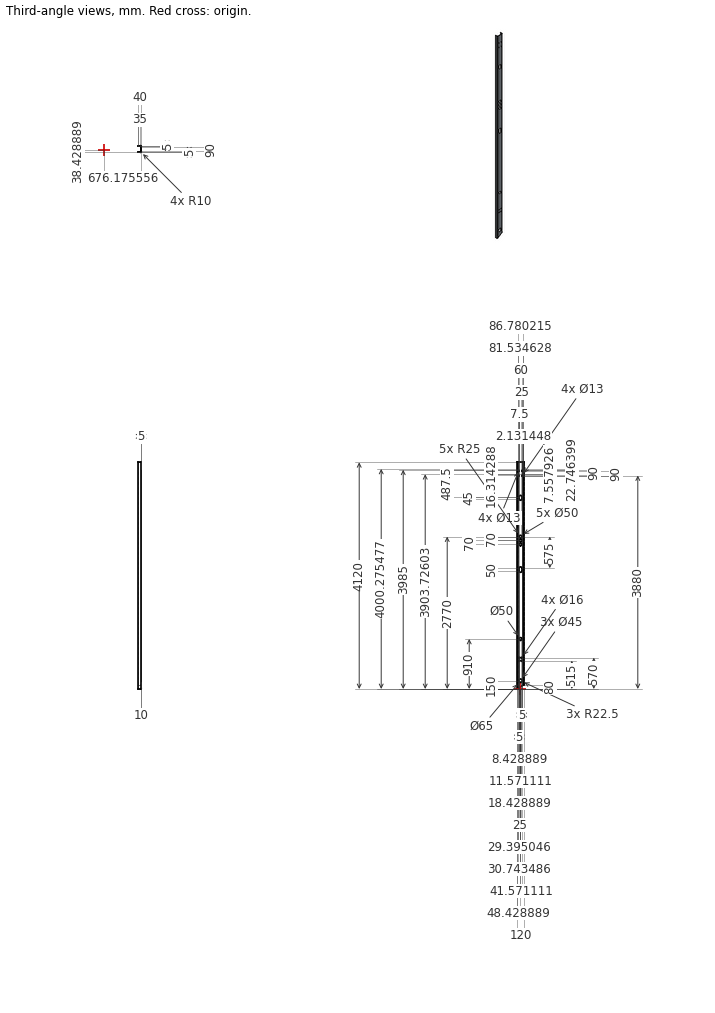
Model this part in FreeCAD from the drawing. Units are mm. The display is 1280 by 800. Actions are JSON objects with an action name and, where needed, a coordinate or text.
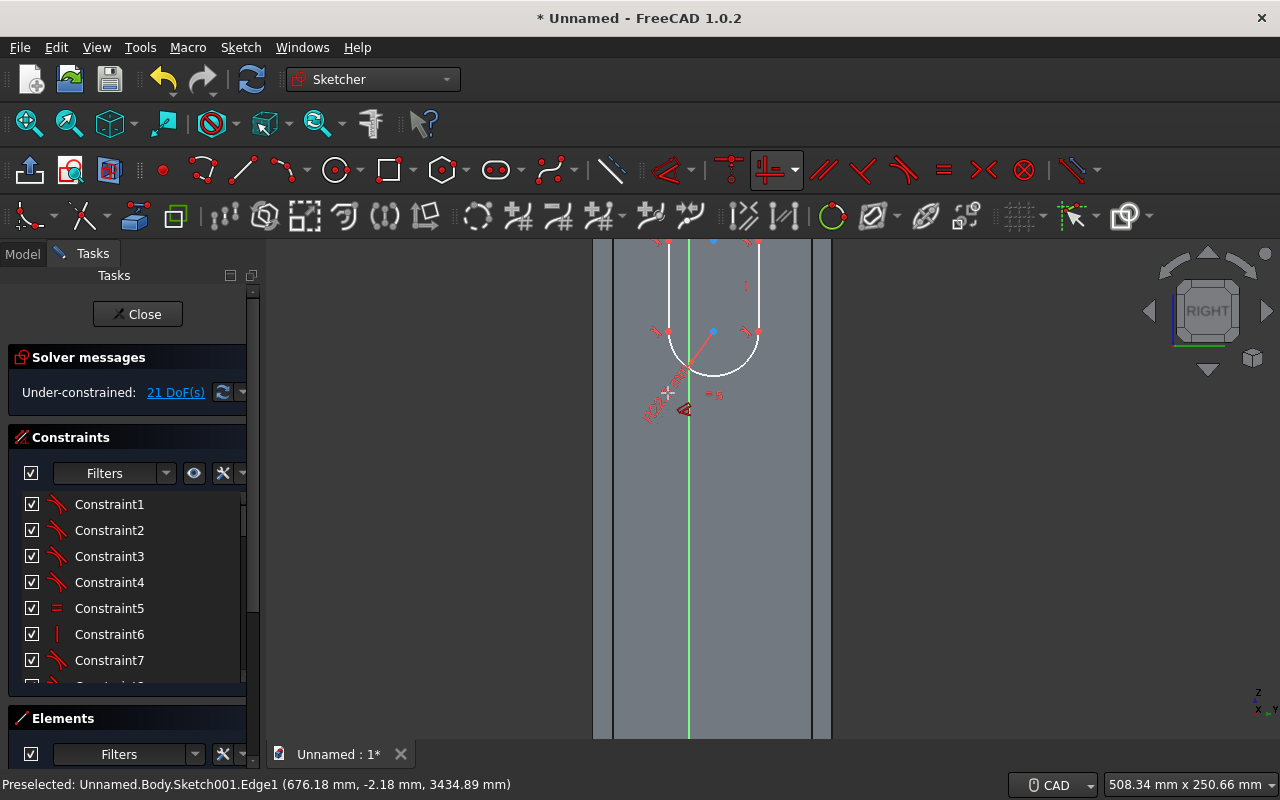
{"action": "scroll", "coordinate": [704, 372], "scroll_direction": "down", "scroll_amount": 16}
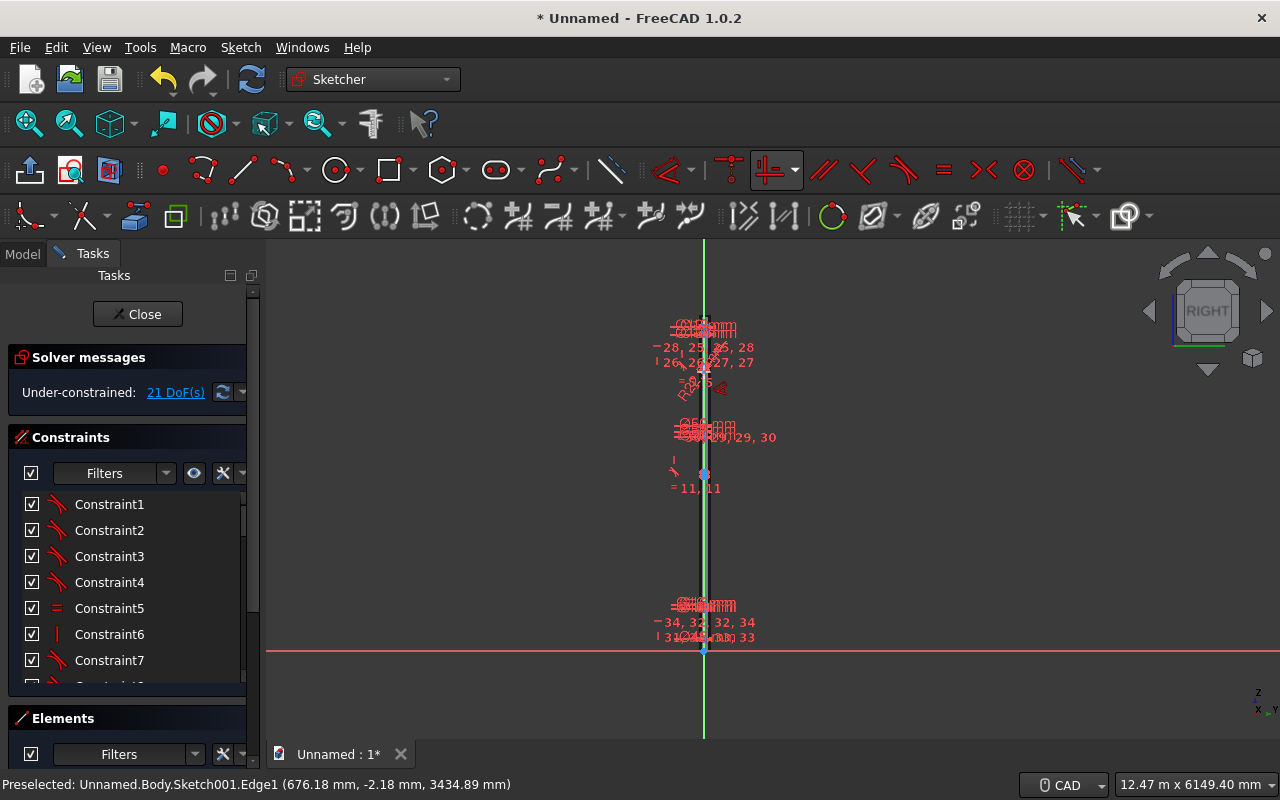
{"action": "scroll", "coordinate": [706, 479], "scroll_direction": "up", "scroll_amount": 15}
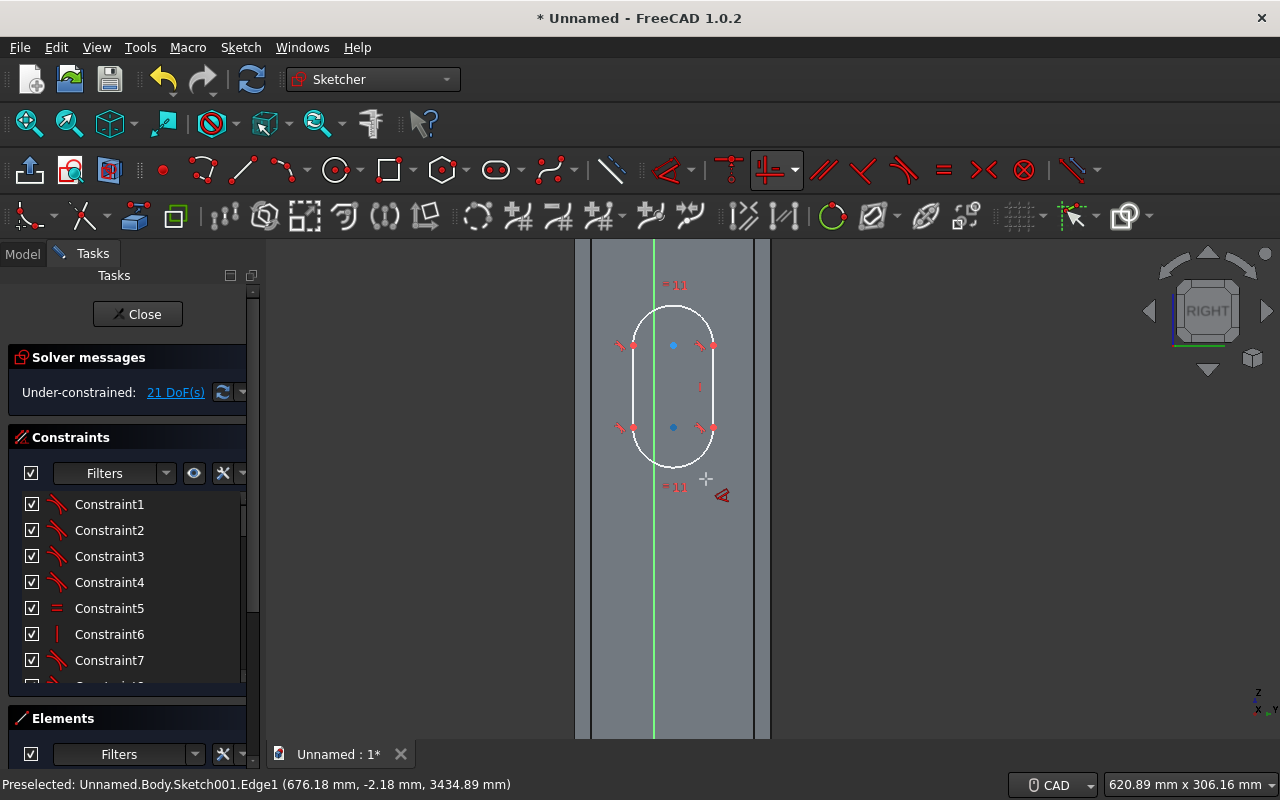
{"action": "left_click", "coordinate": [697, 460]}
{"action": "left_click", "coordinate": [716, 486]}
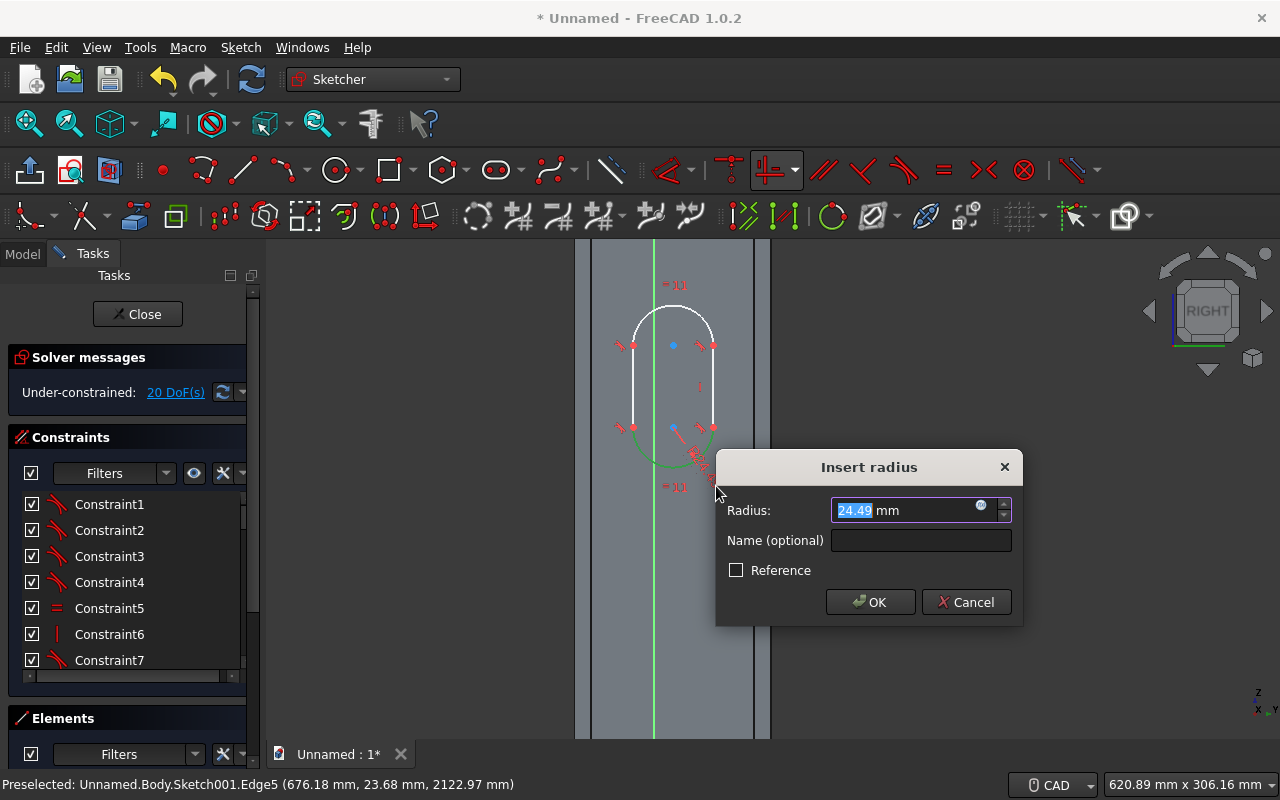
{"action": "type", "text": "25"}
{"action": "key", "text": "Return"}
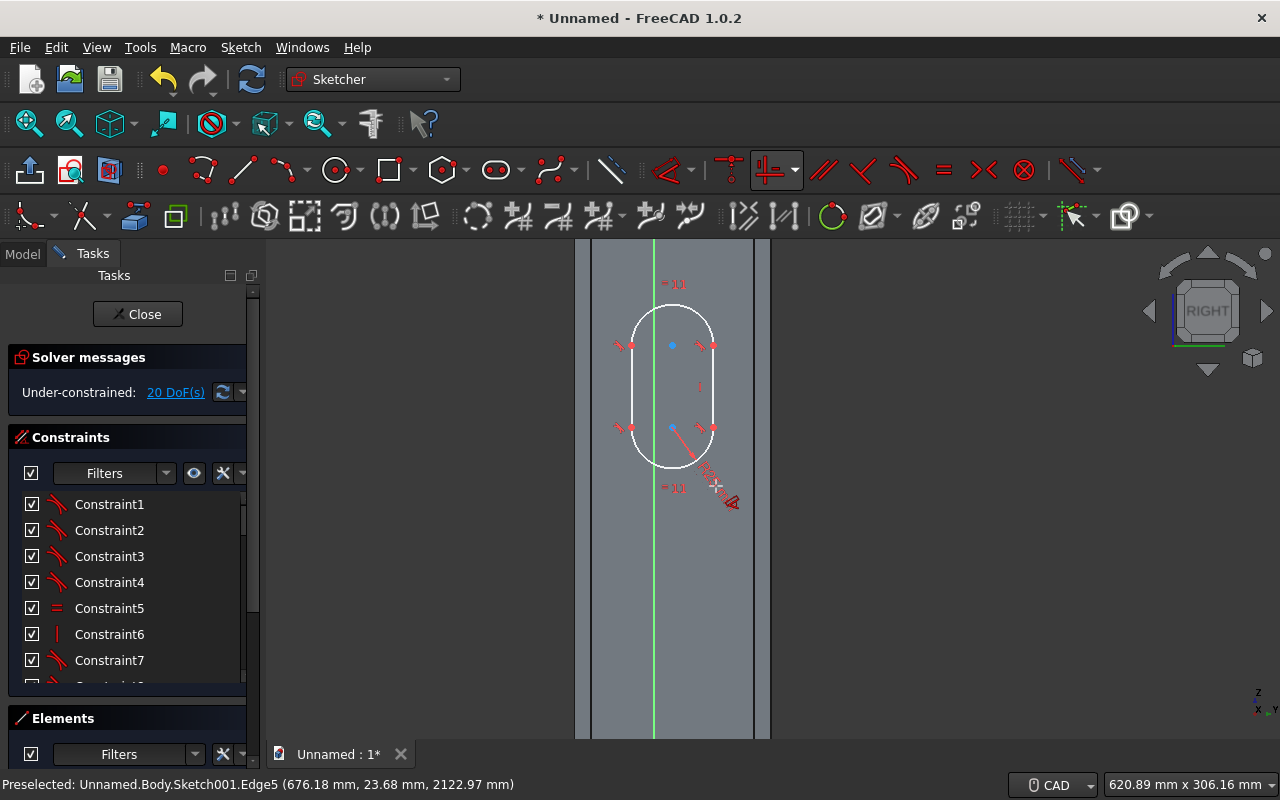
{"action": "scroll", "coordinate": [706, 479], "scroll_direction": "down", "scroll_amount": 15}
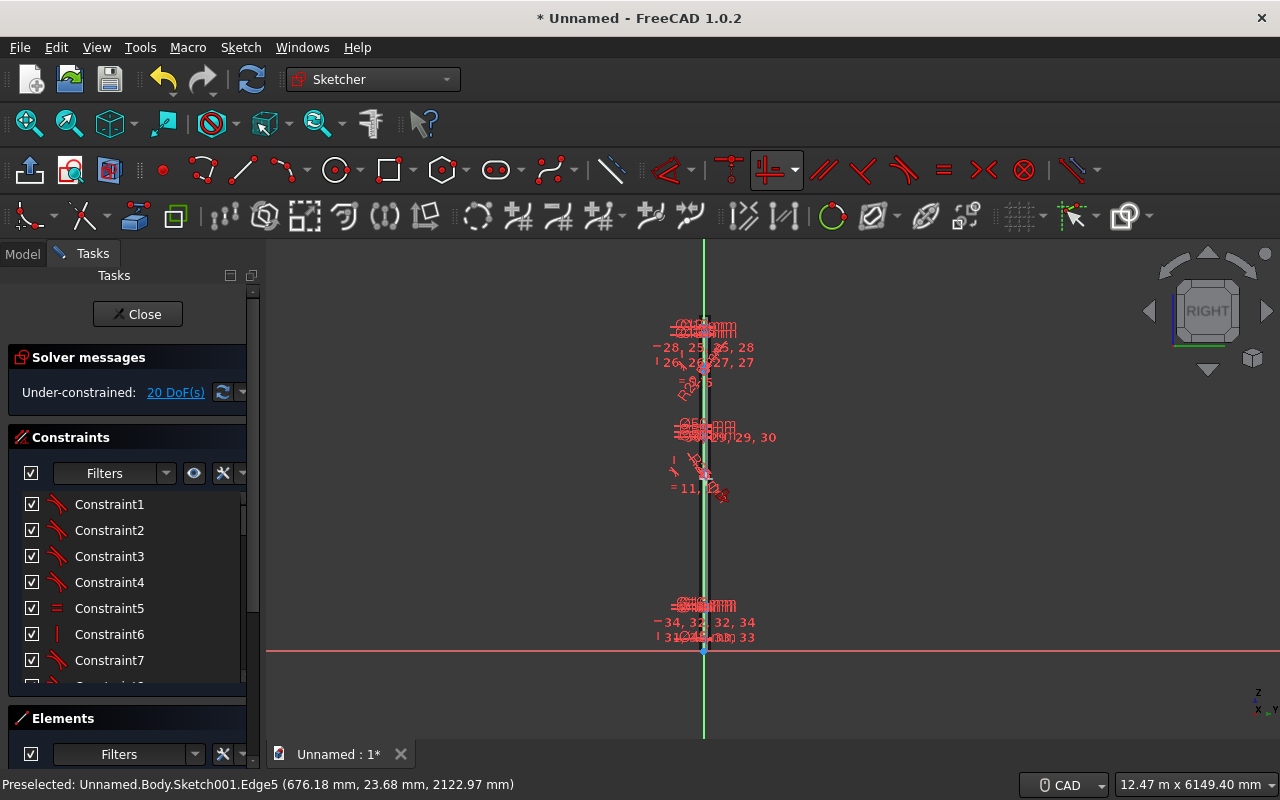
{"action": "scroll", "coordinate": [703, 369], "scroll_direction": "up", "scroll_amount": 14}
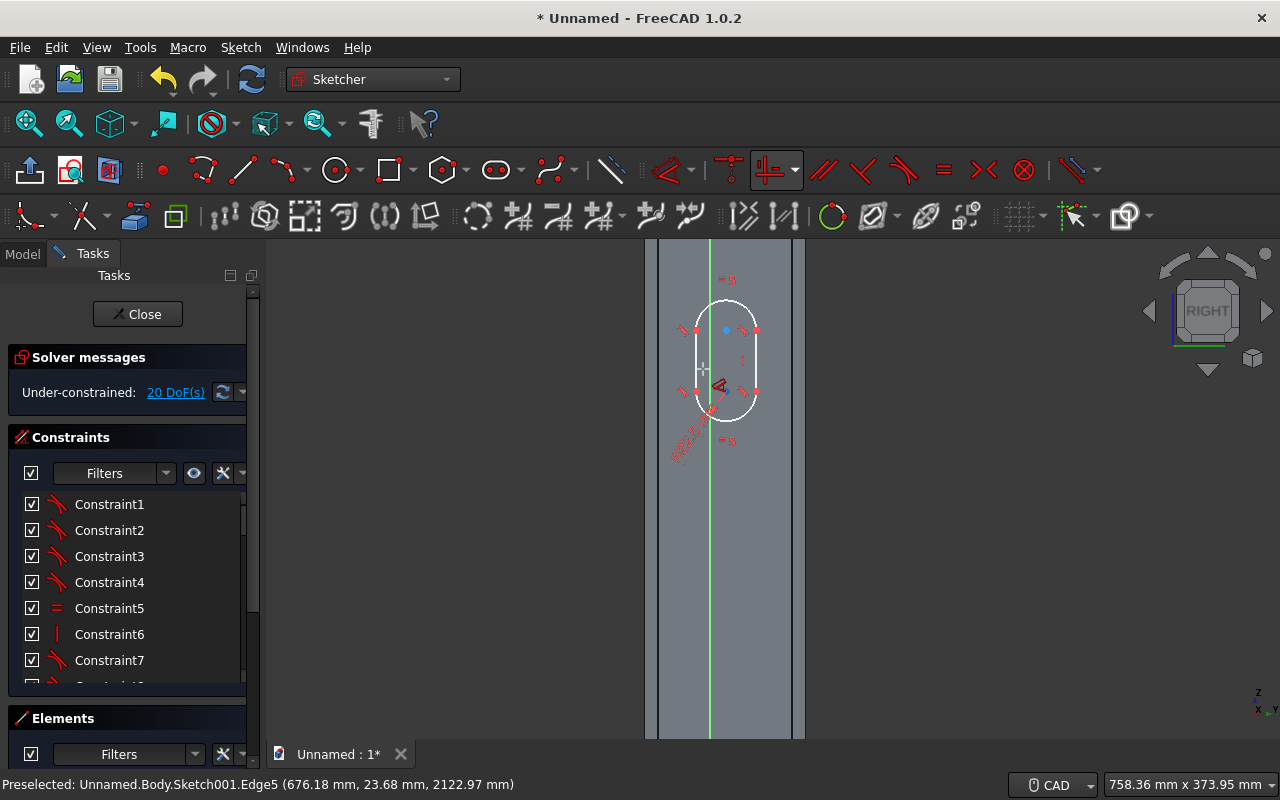
{"action": "left_click", "coordinate": [696, 373]}
{"action": "left_click", "coordinate": [662, 361]}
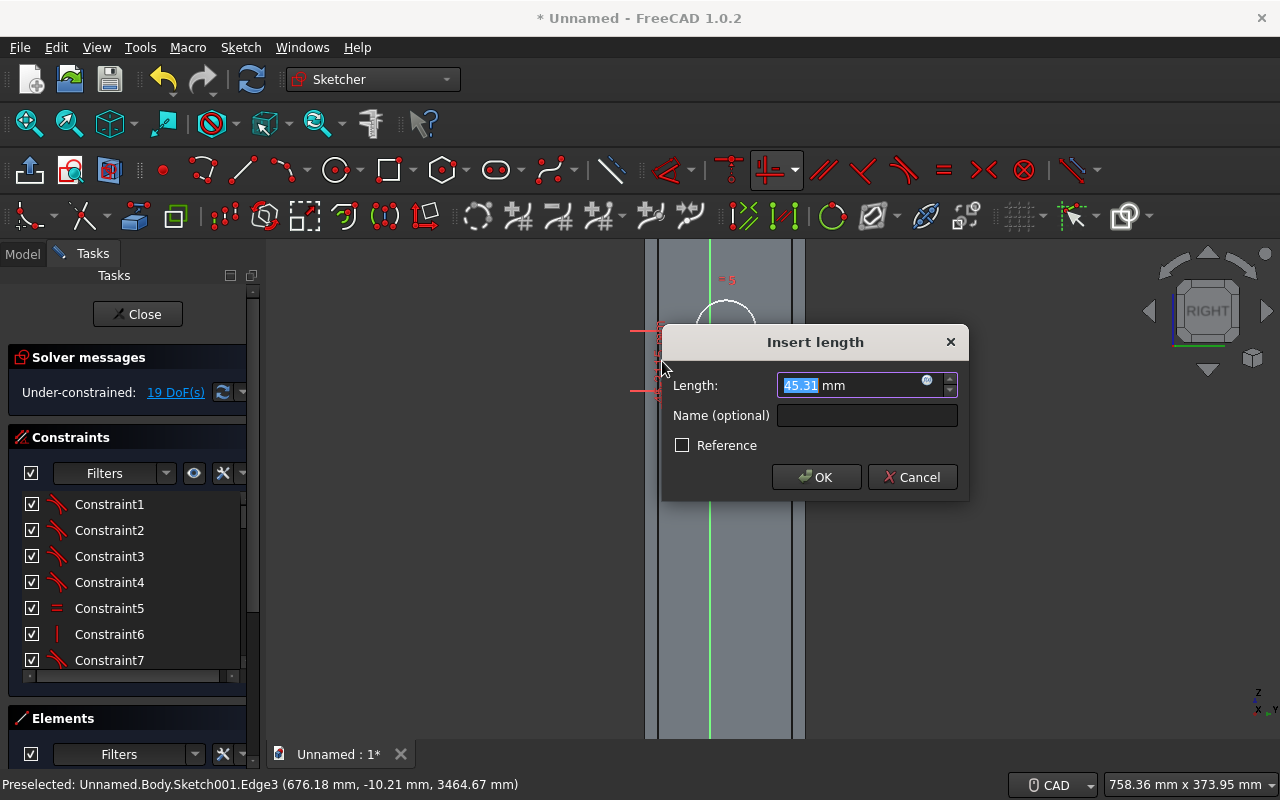
{"action": "type", "text": "45"}
{"action": "key", "text": "Return"}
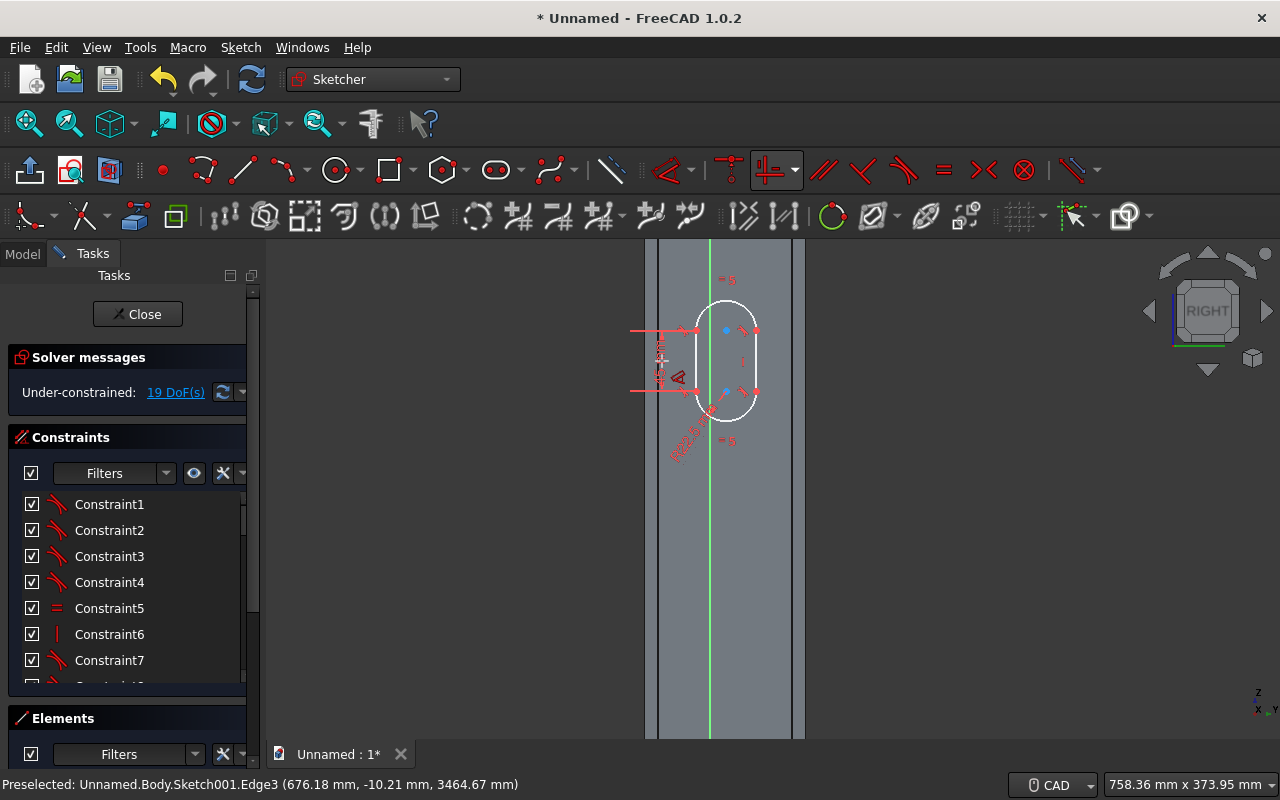
{"action": "scroll", "coordinate": [703, 369], "scroll_direction": "down", "scroll_amount": 14}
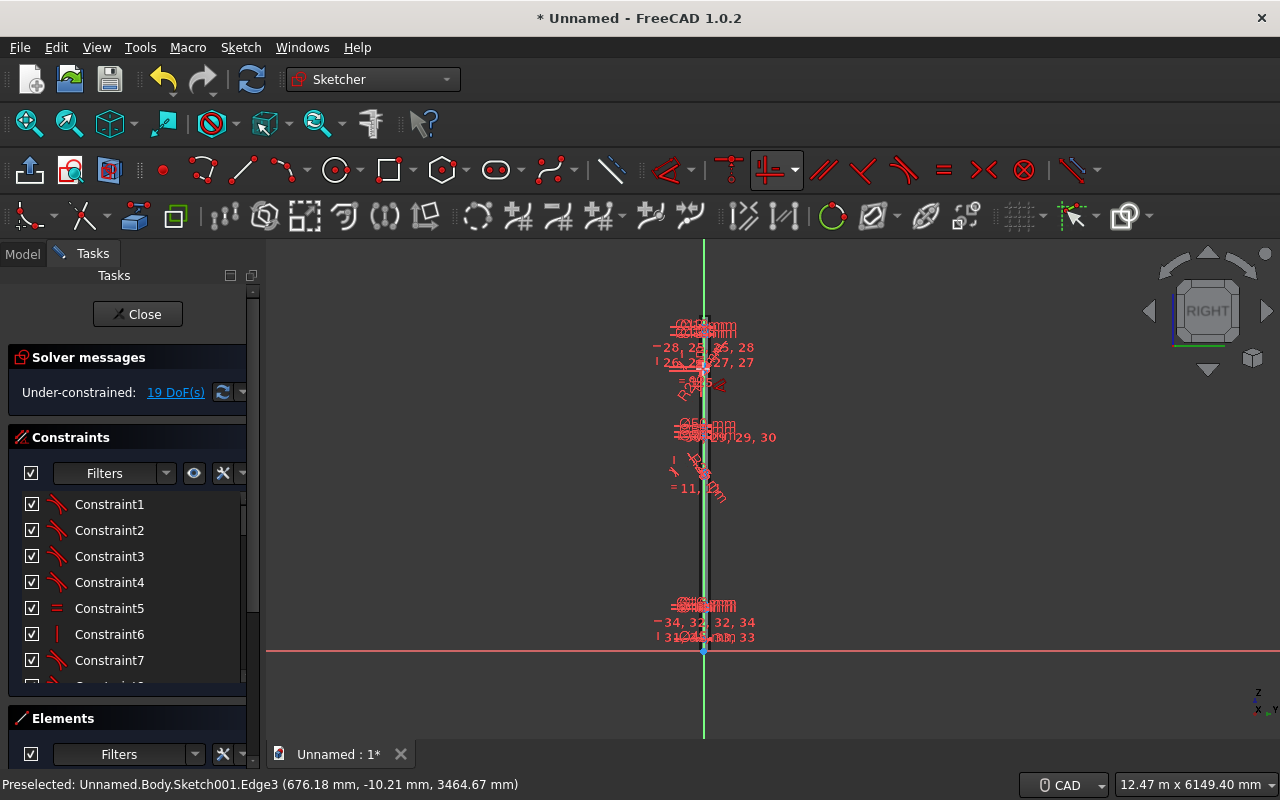
{"action": "scroll", "coordinate": [703, 476], "scroll_direction": "up", "scroll_amount": 13}